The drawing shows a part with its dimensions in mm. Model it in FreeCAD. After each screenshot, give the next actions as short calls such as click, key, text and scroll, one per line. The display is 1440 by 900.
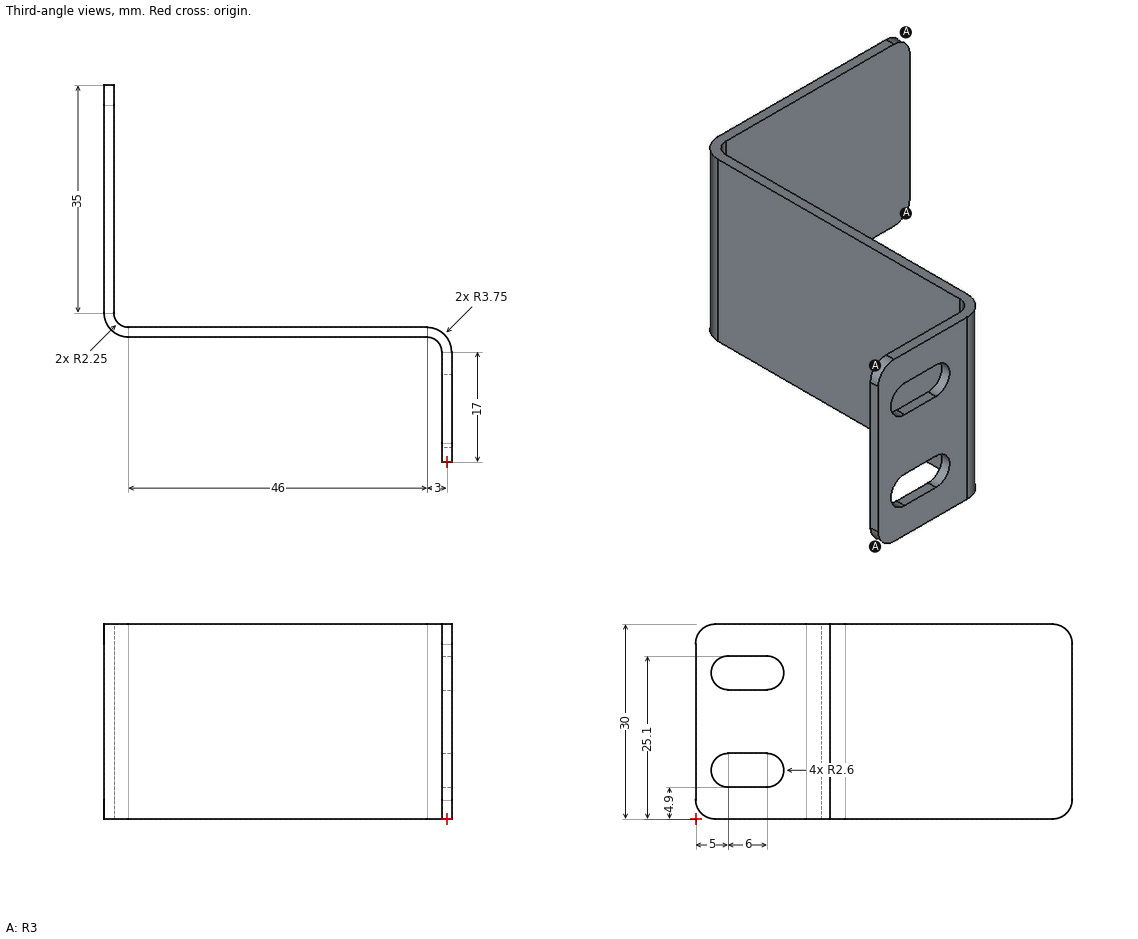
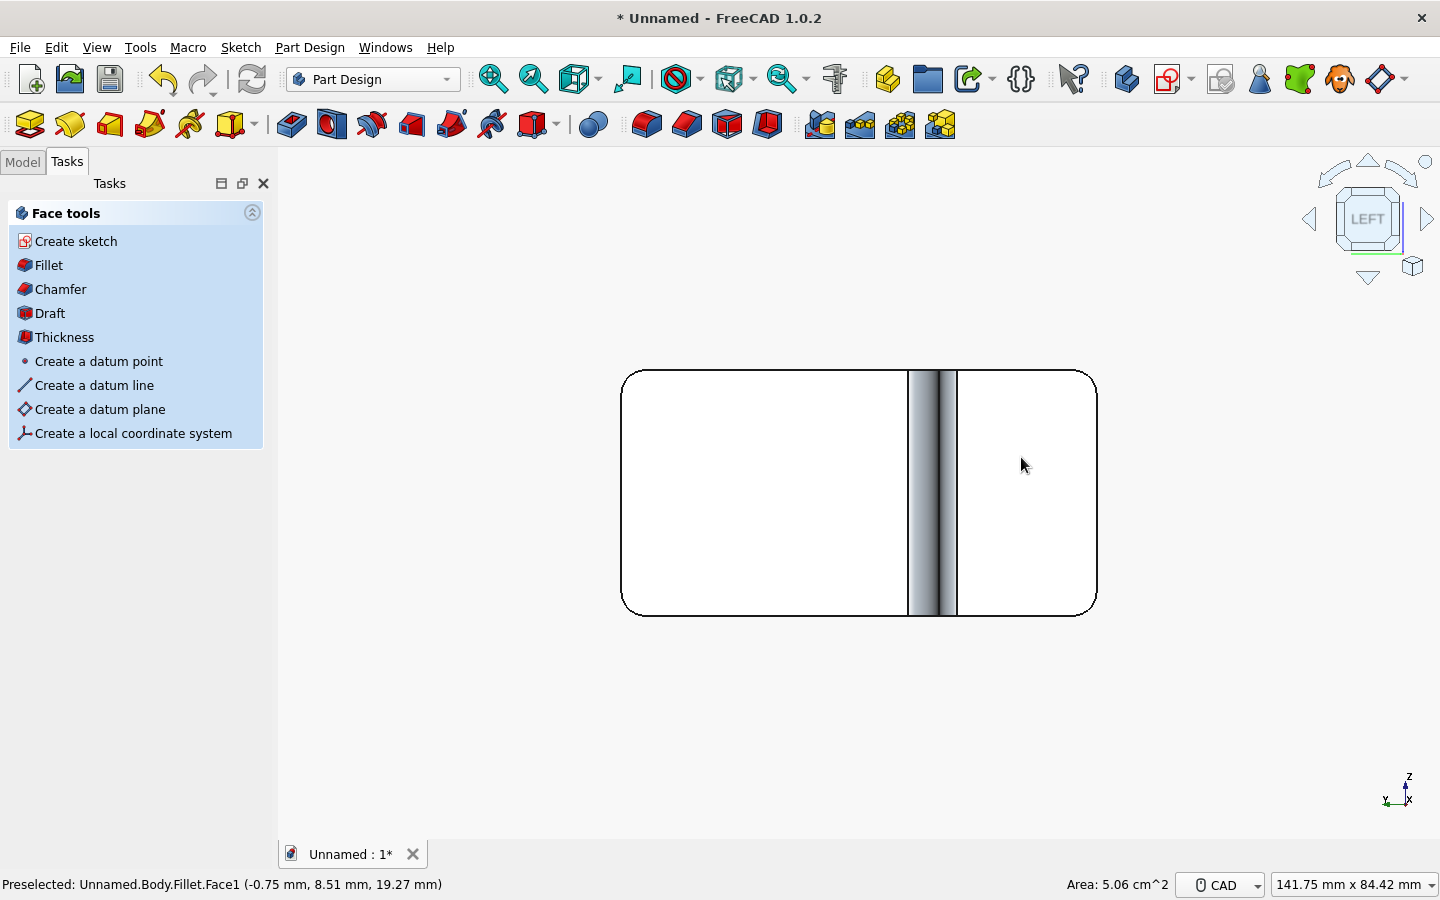
click(1168, 80)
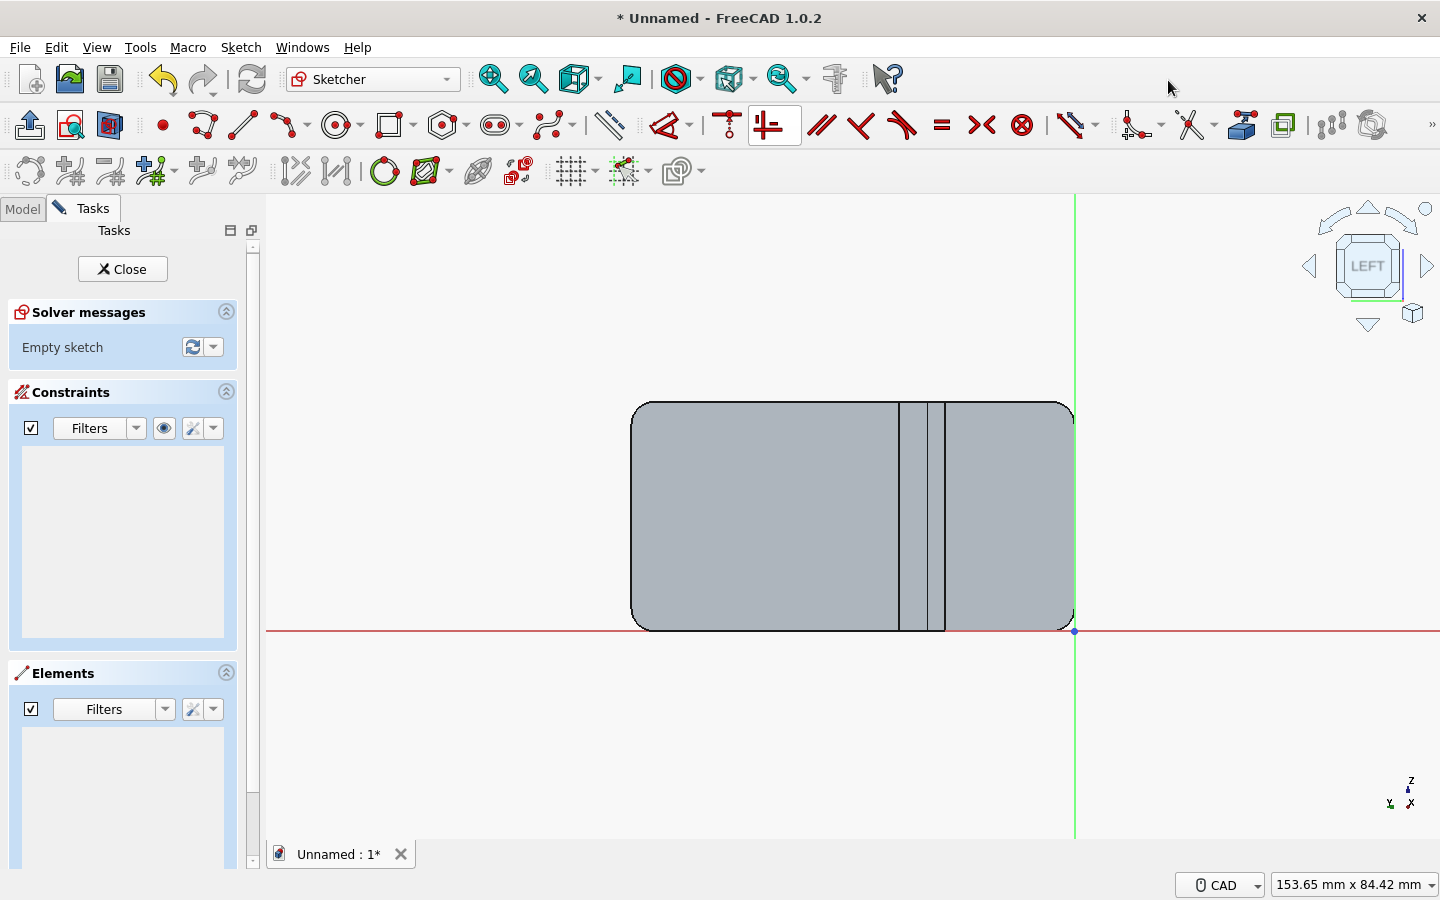
scroll(1217, 550, up, 4)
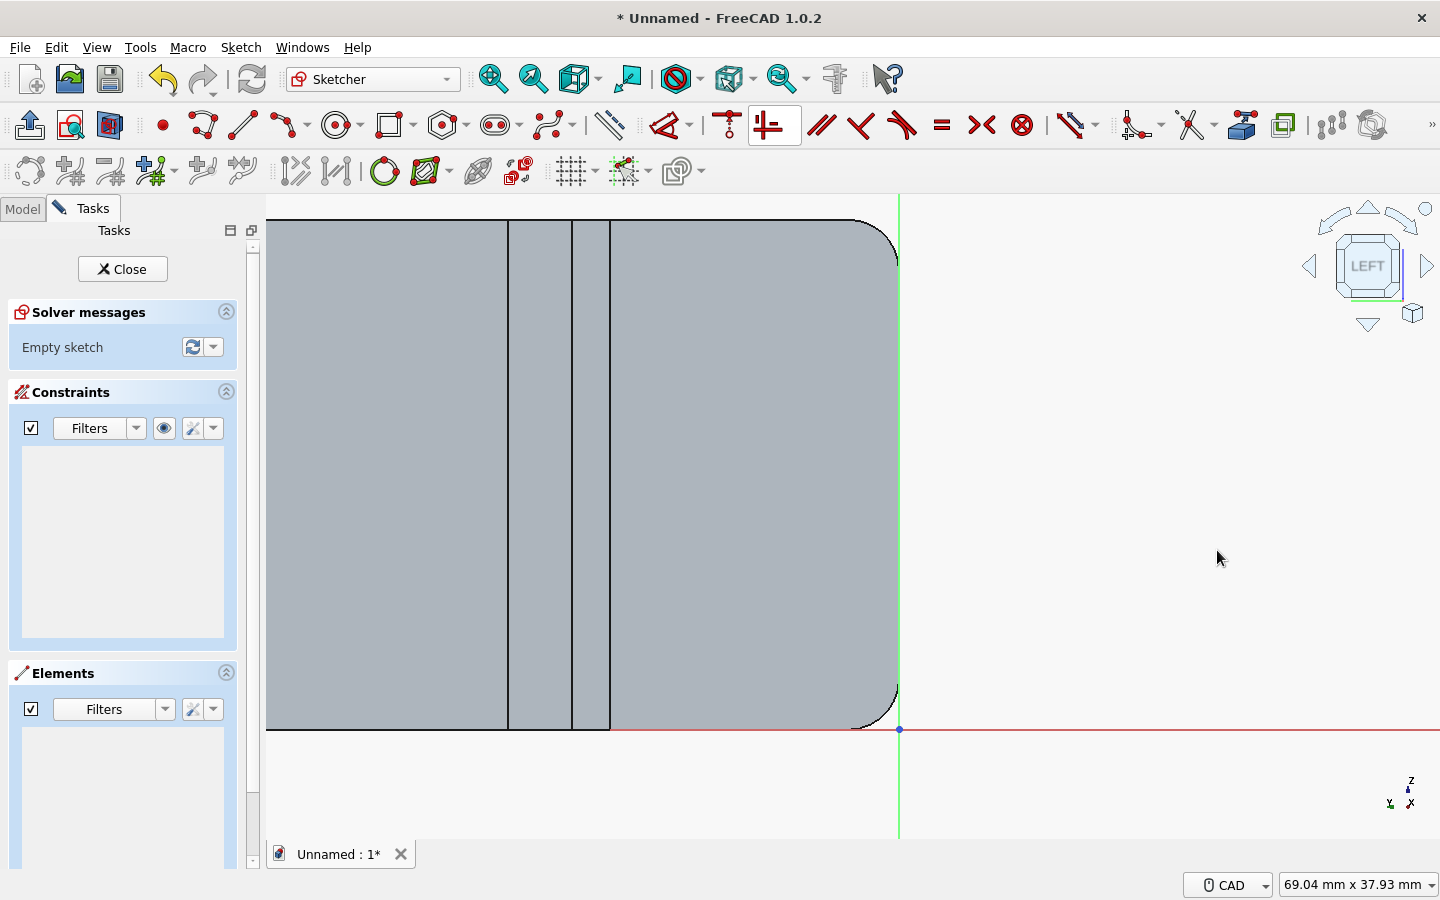
key(g)
key(s)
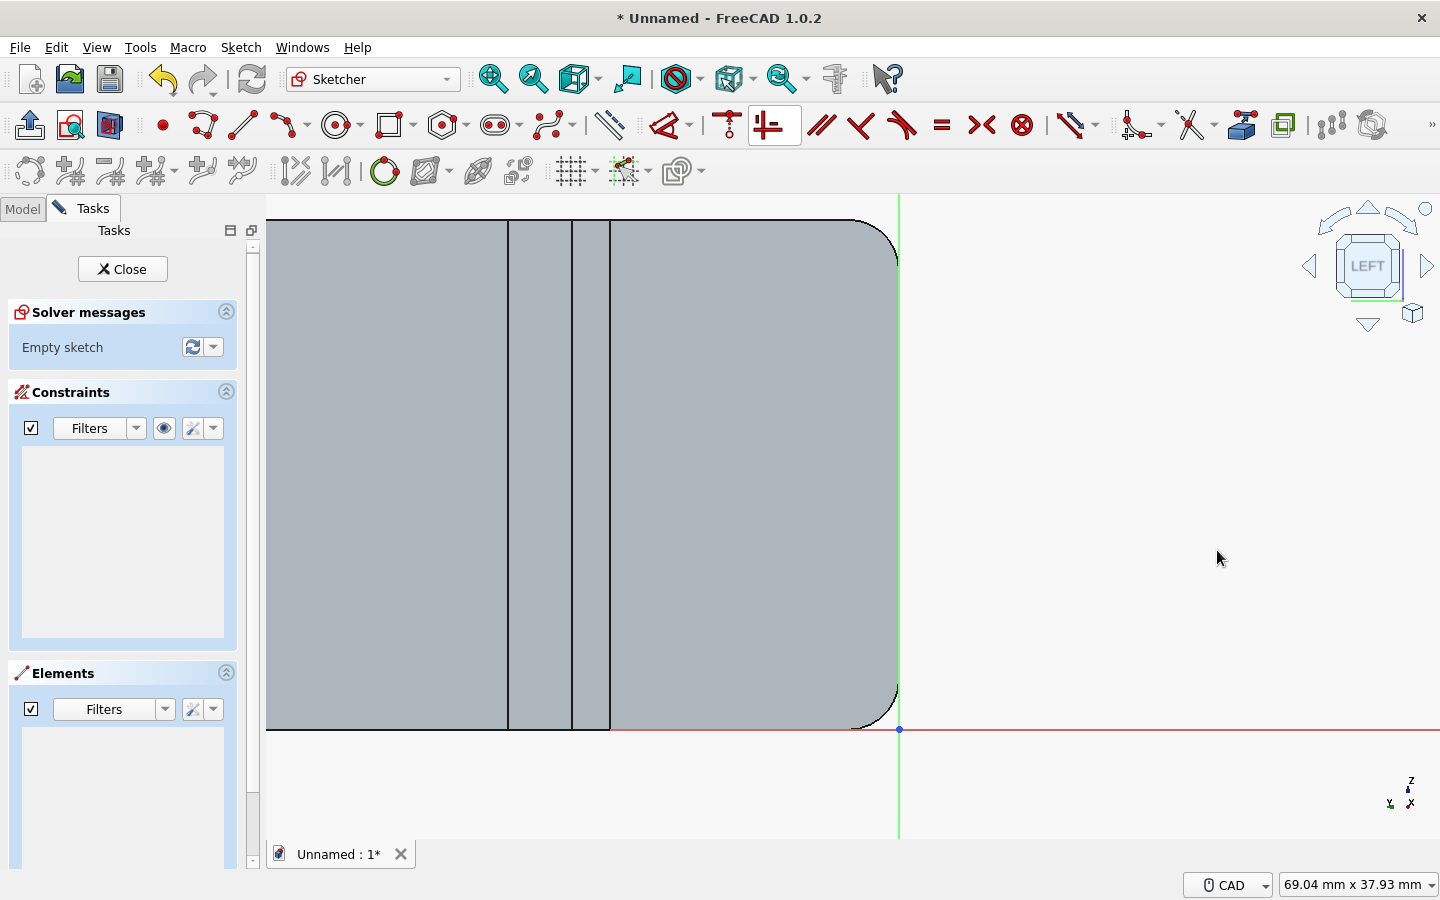
click(712, 602)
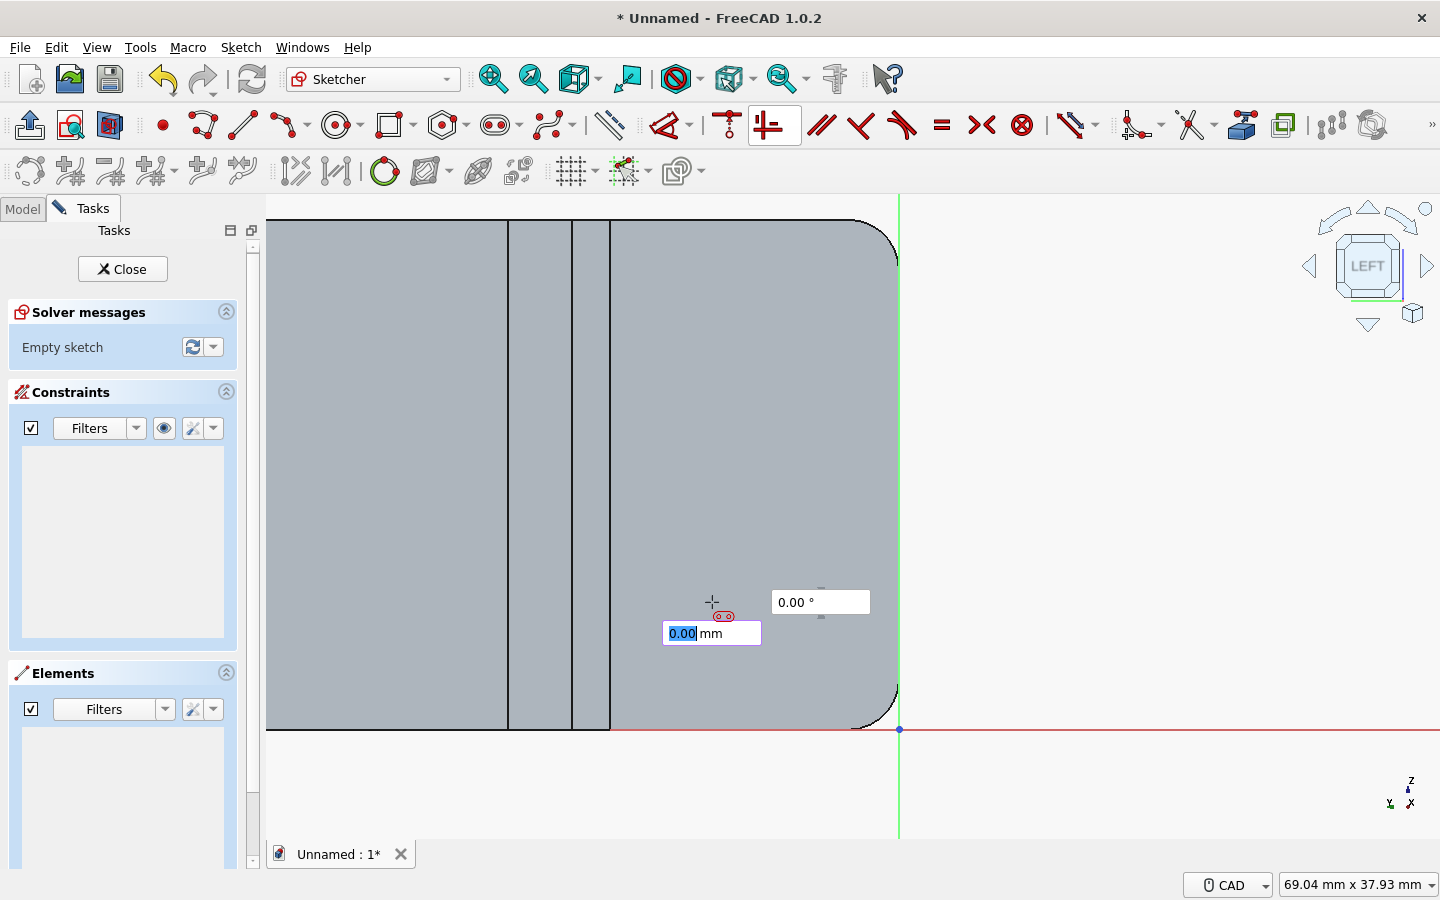
click(814, 602)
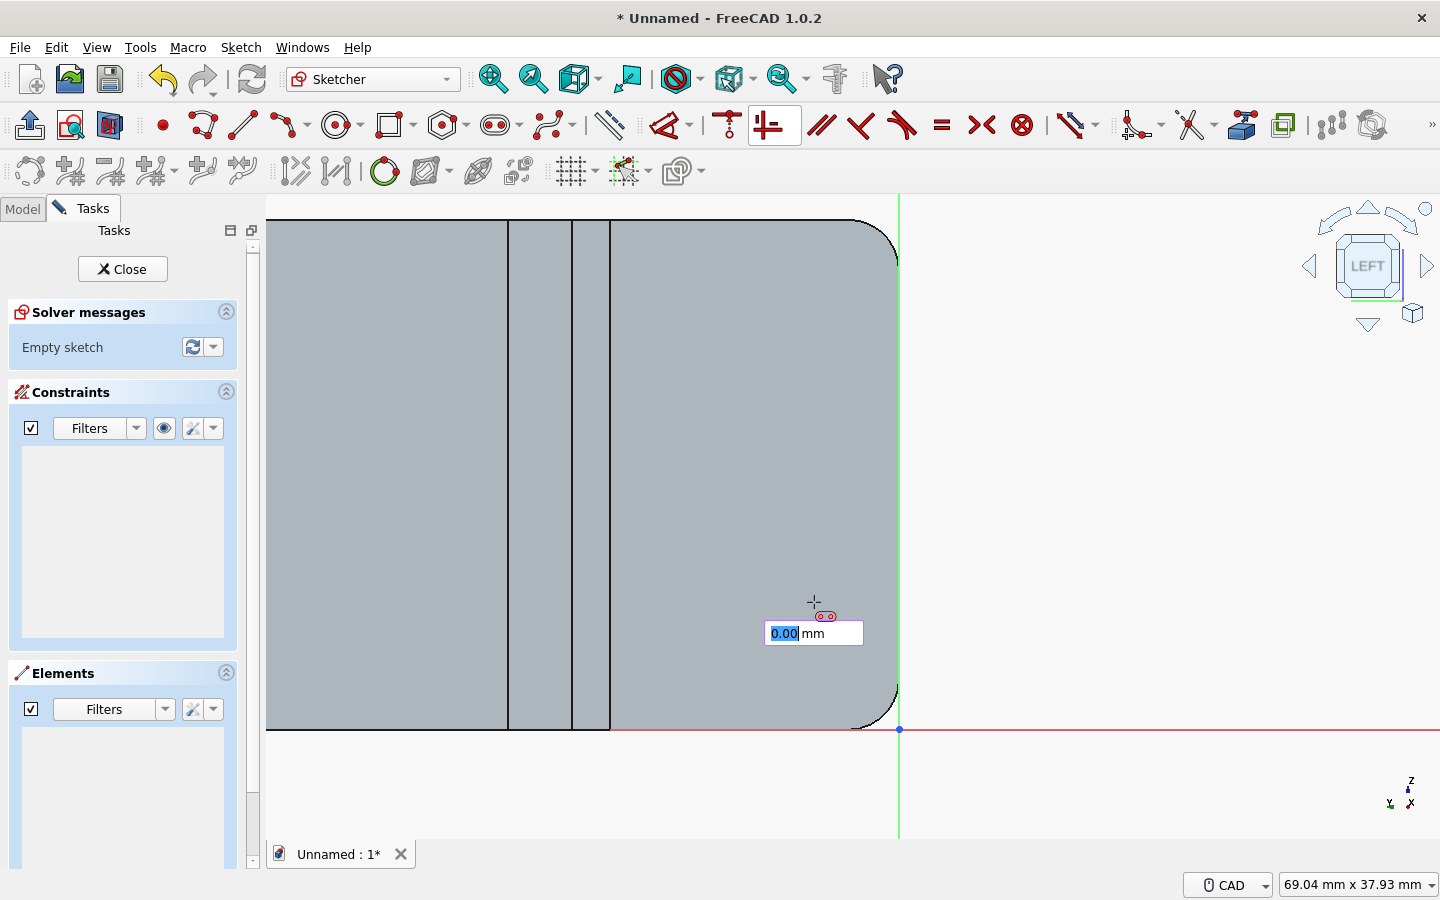
click(763, 558)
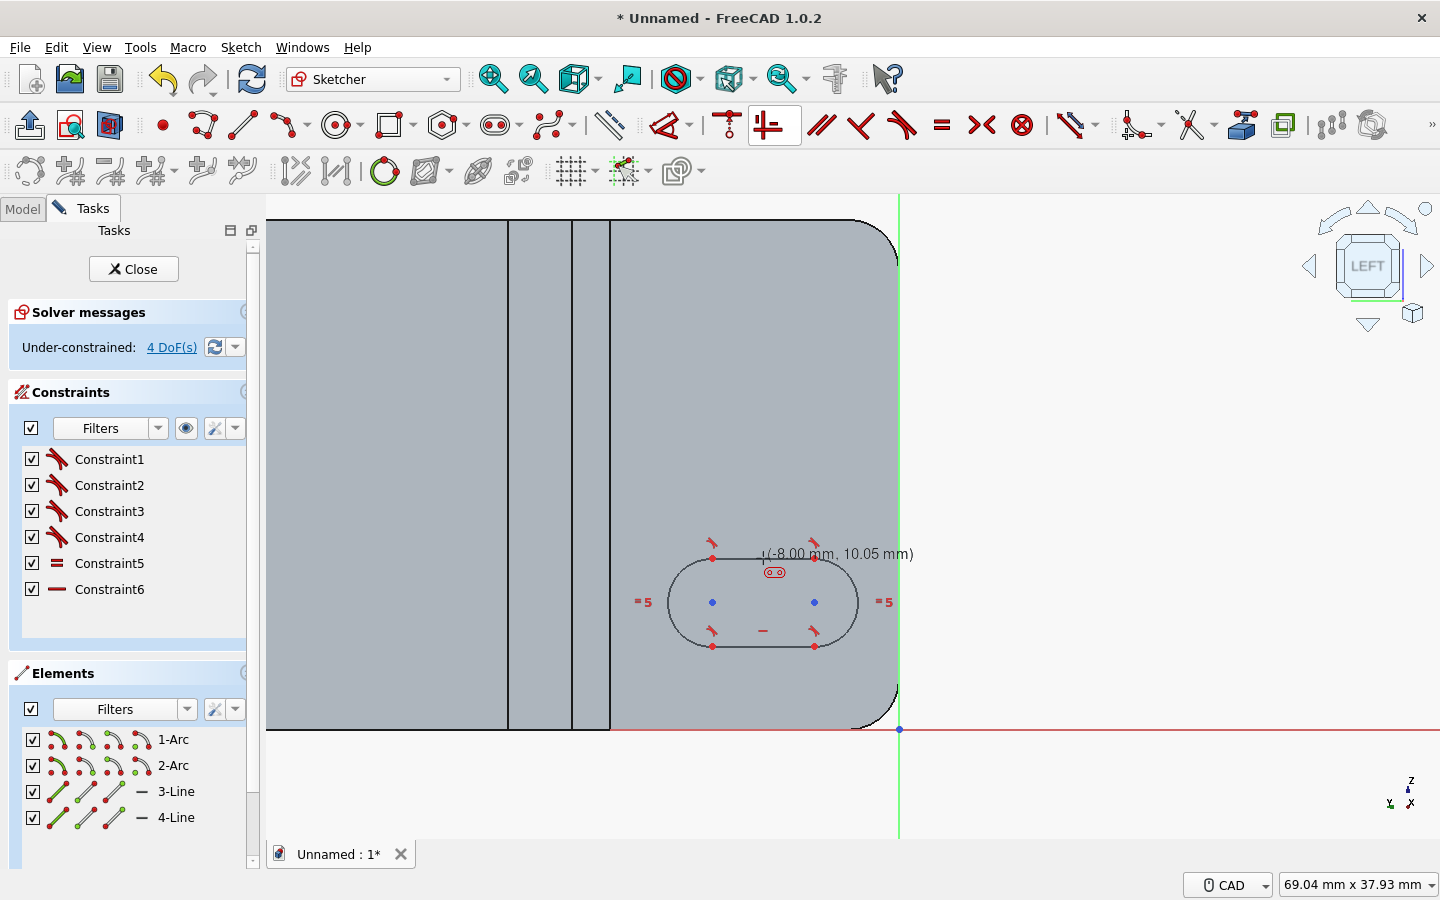
click(712, 347)